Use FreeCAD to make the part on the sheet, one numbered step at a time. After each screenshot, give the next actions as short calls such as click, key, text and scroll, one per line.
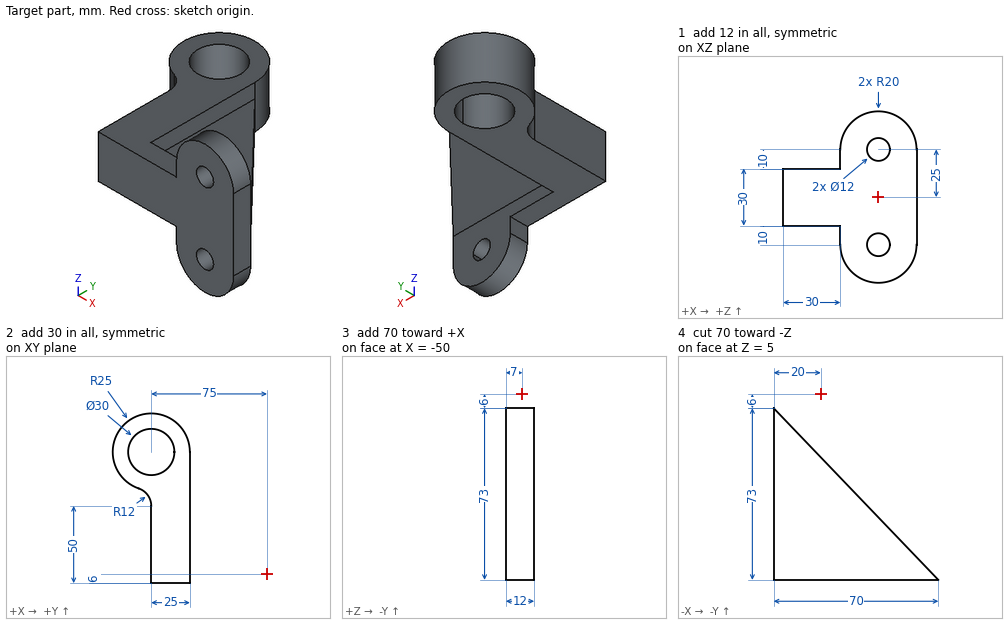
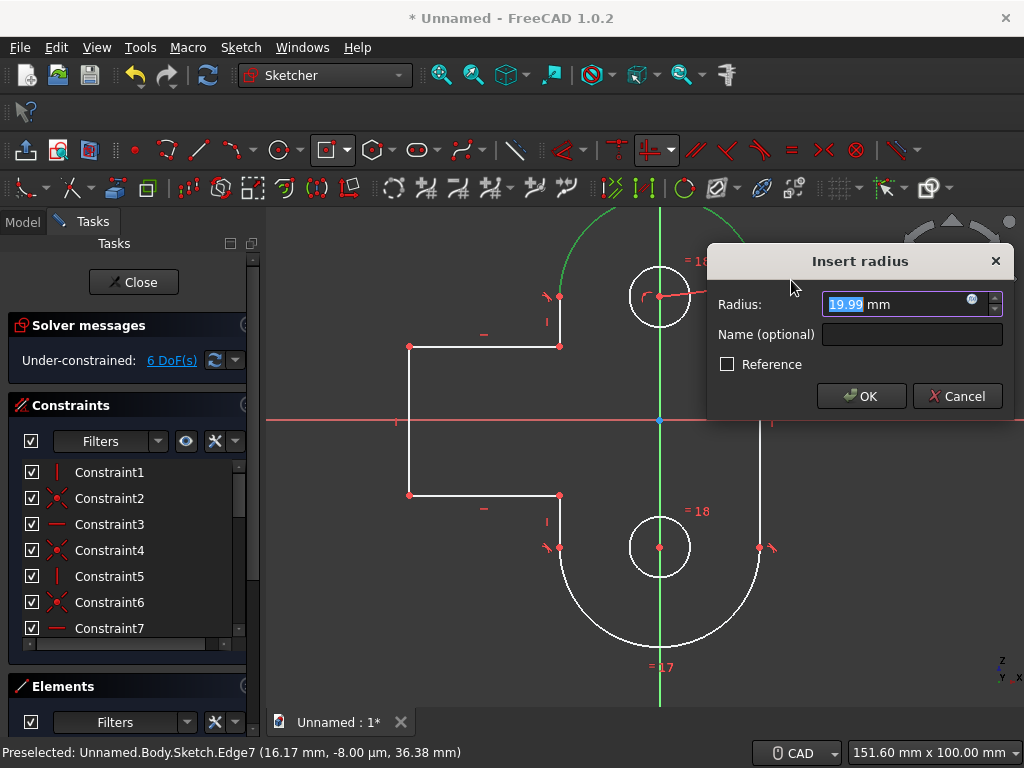
text(20)
key(Return)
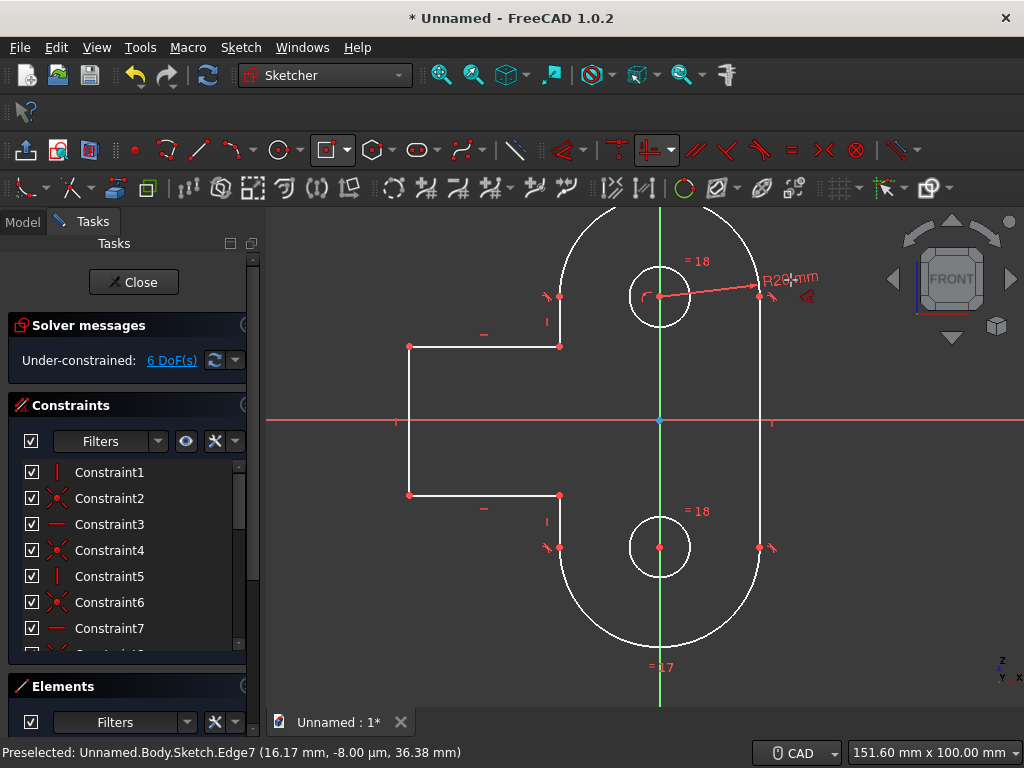
click(681, 275)
click(703, 252)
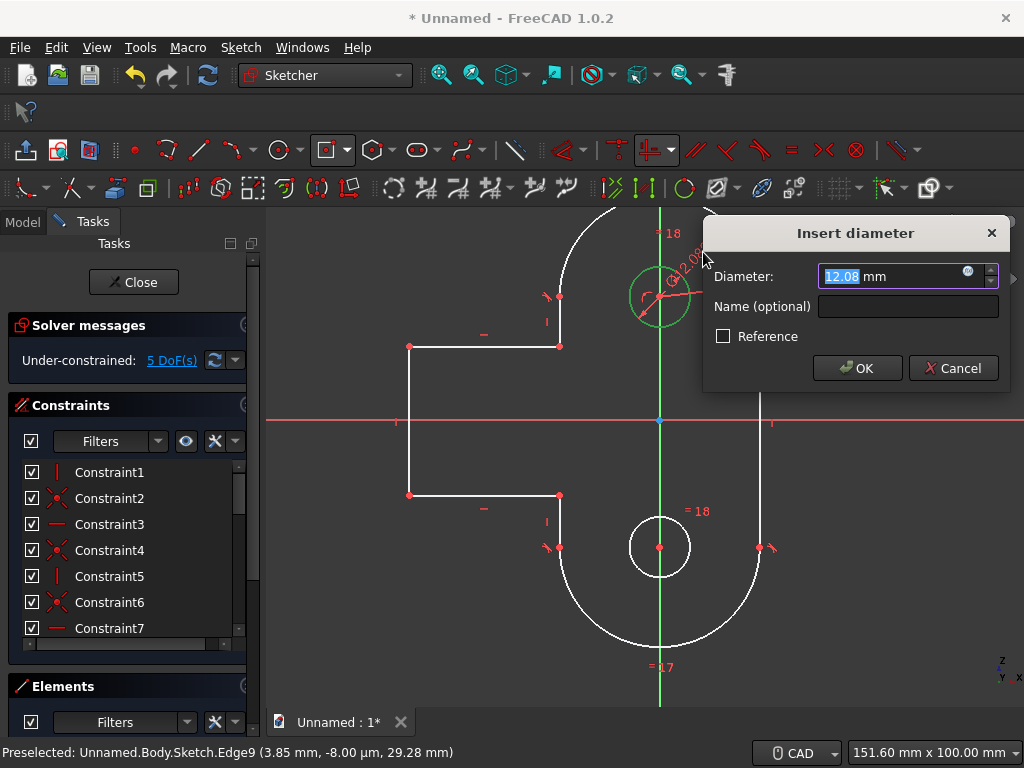
text(12)
key(Return)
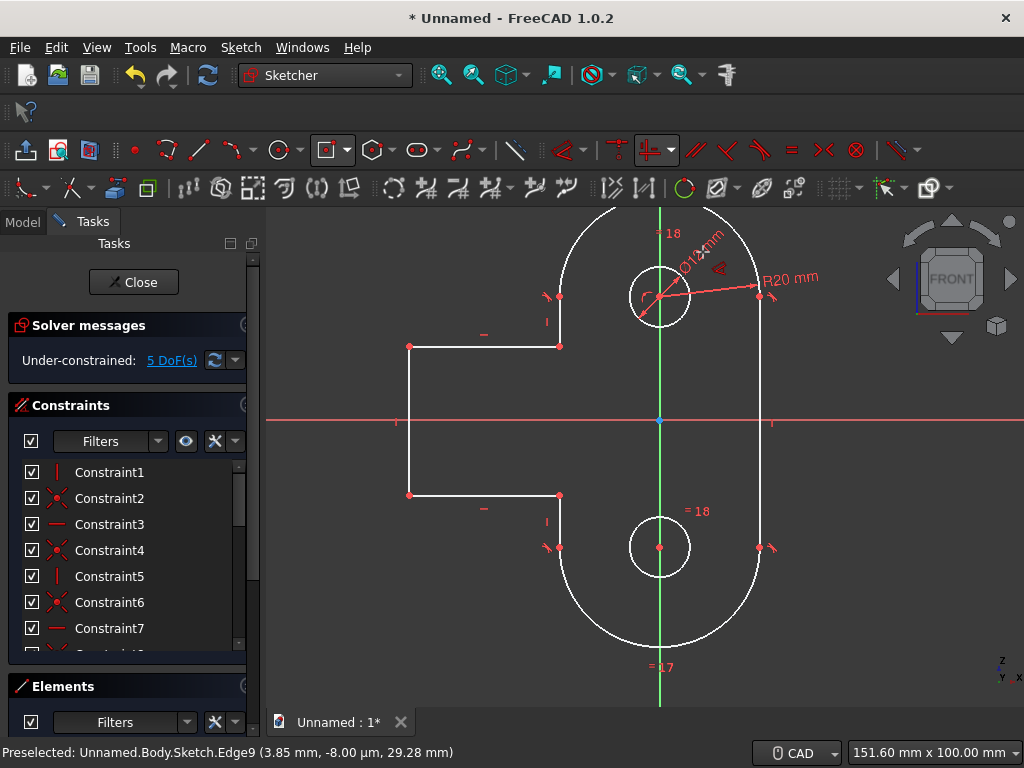
click(560, 532)
click(526, 522)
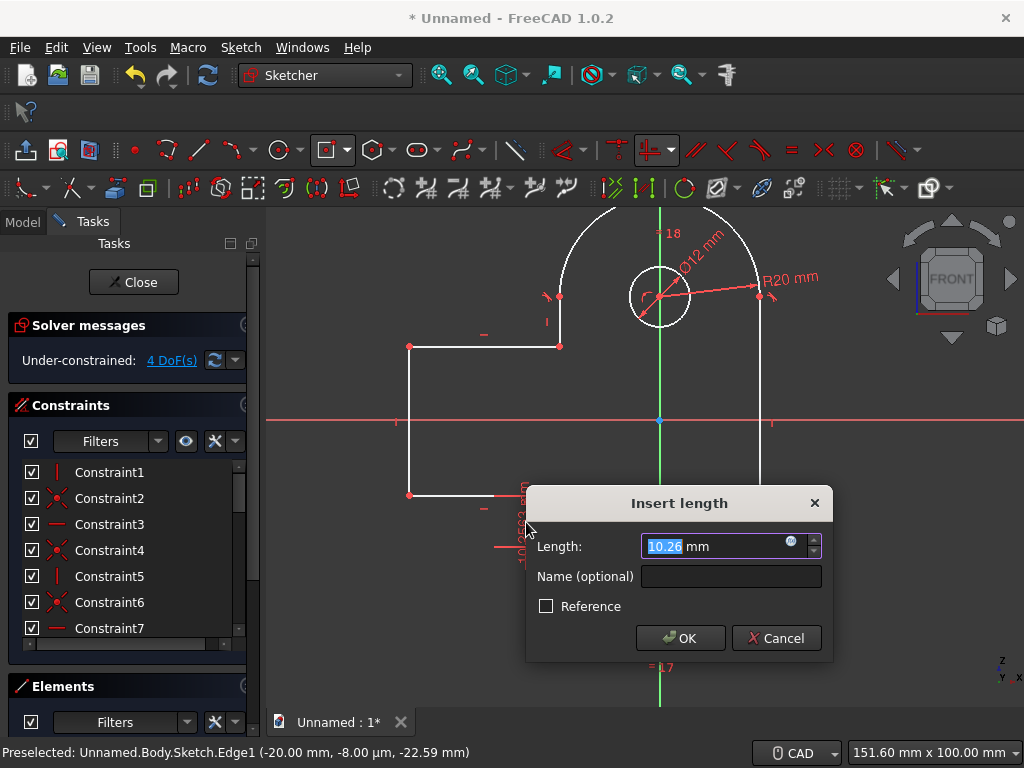
text(10)
key(Return)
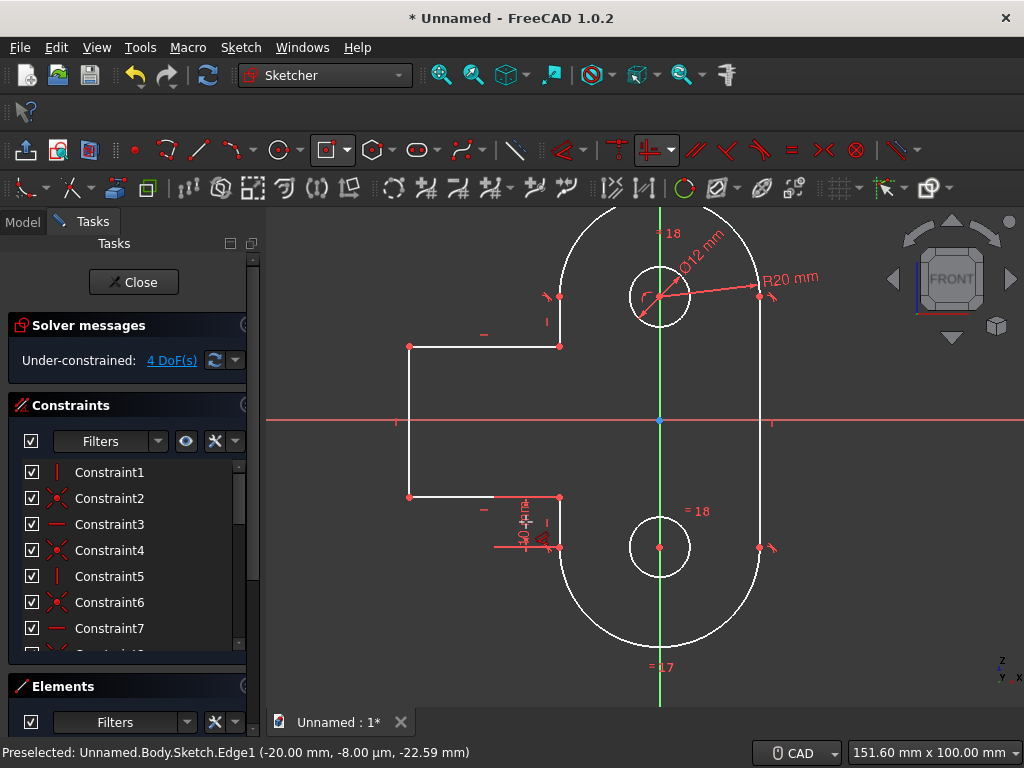
click(515, 497)
click(450, 531)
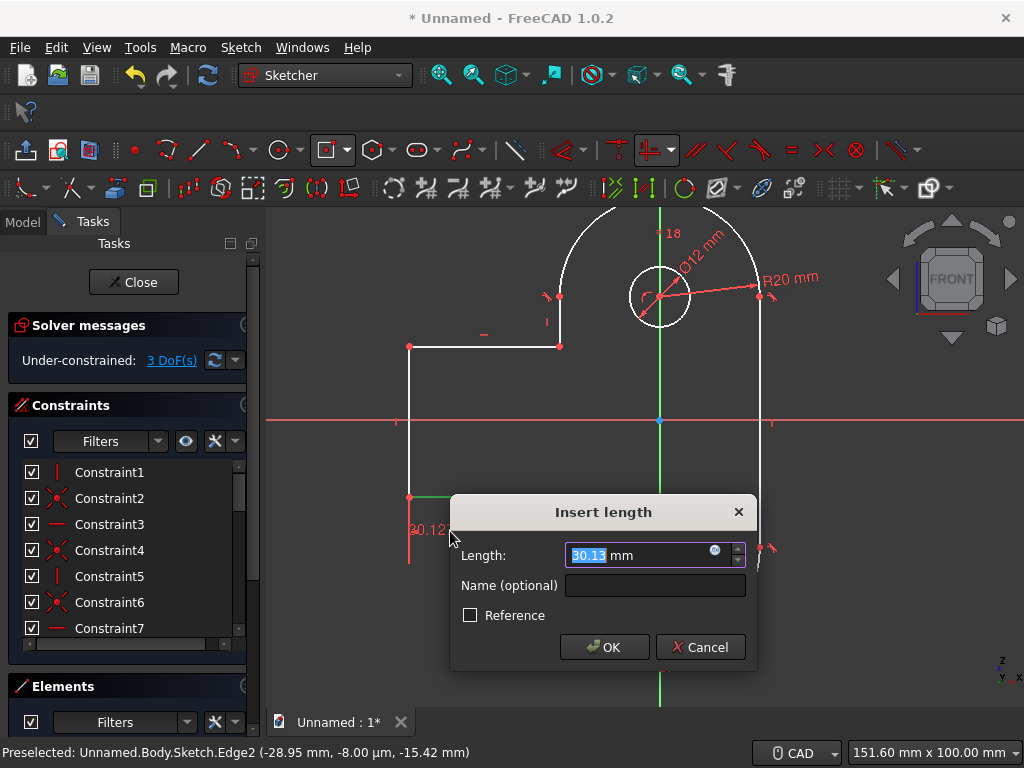
text(30)
key(Return)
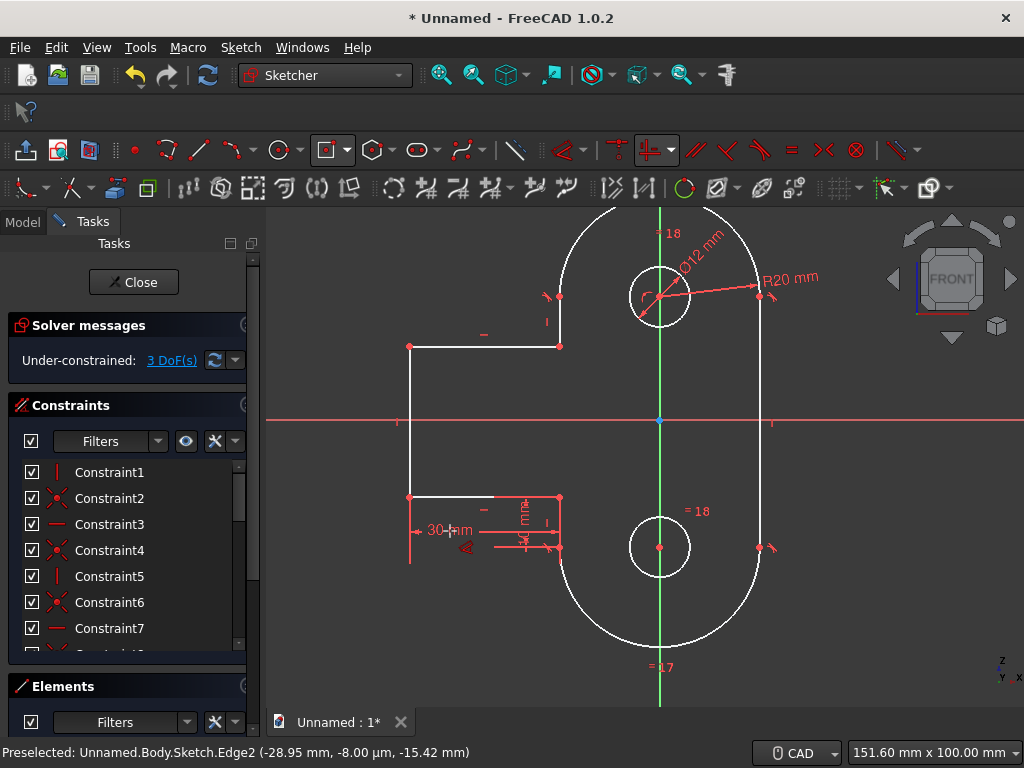
click(410, 452)
click(376, 387)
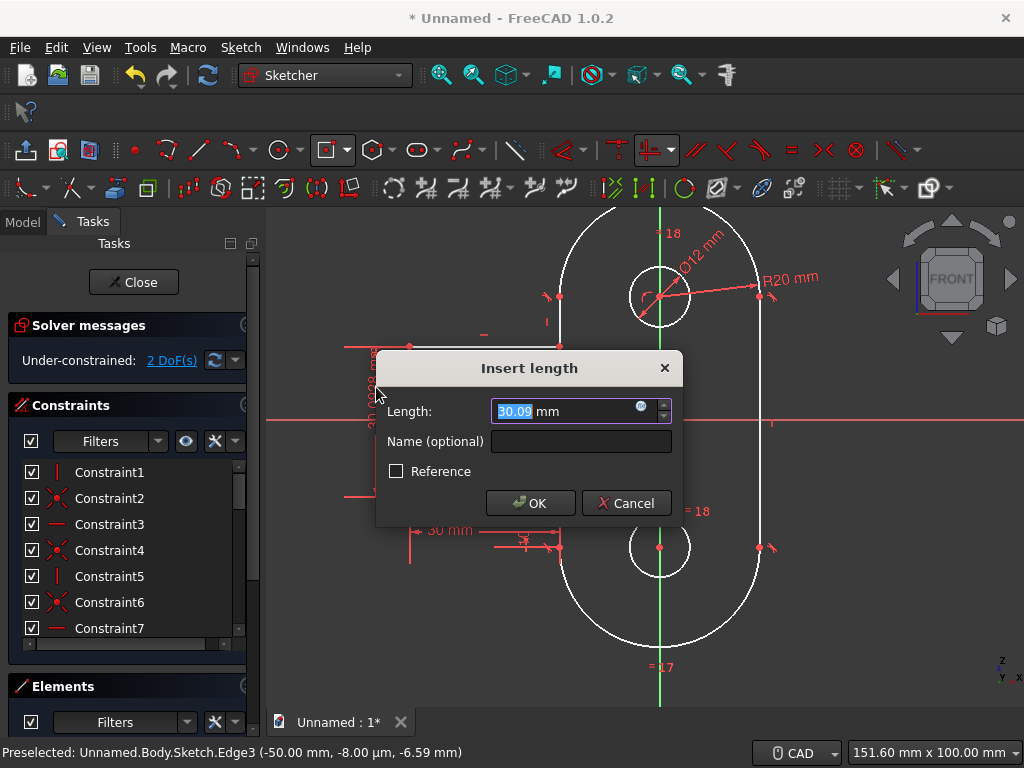
text(30)
key(Return)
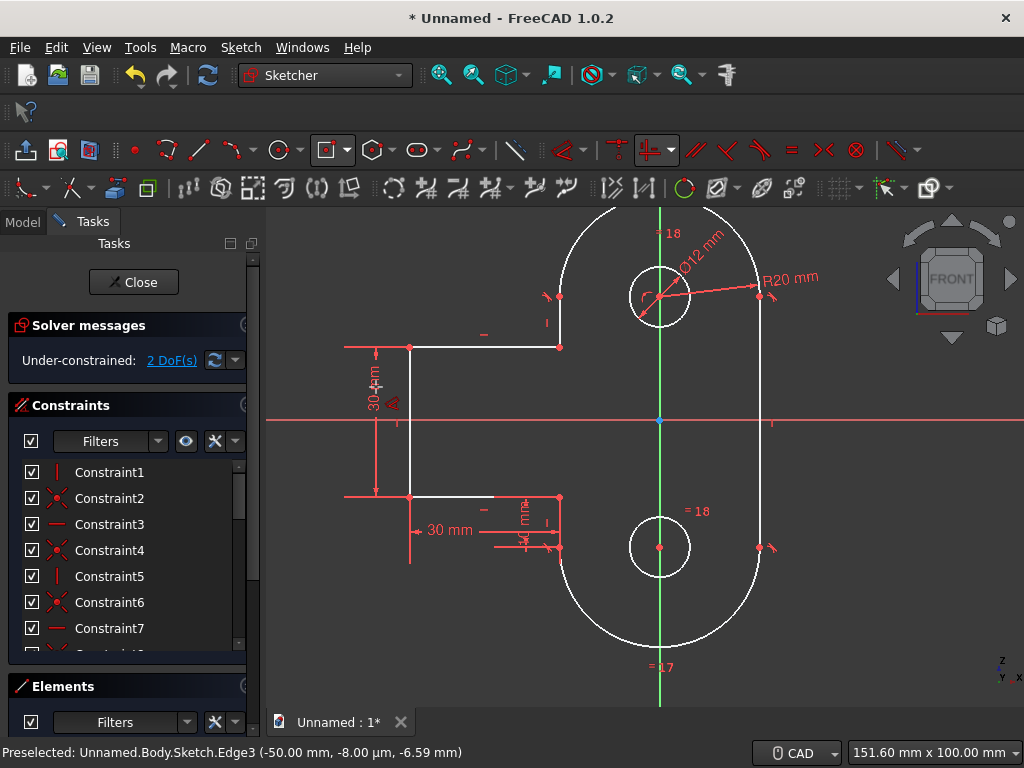
click(560, 332)
click(526, 322)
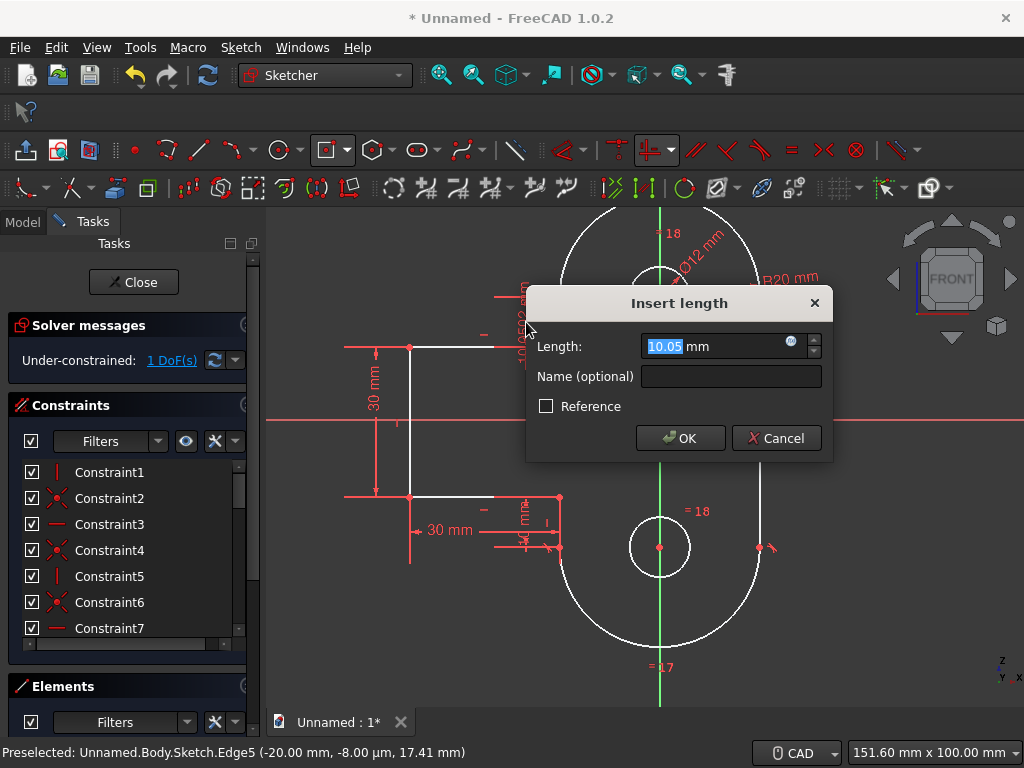
text(10)
key(Return)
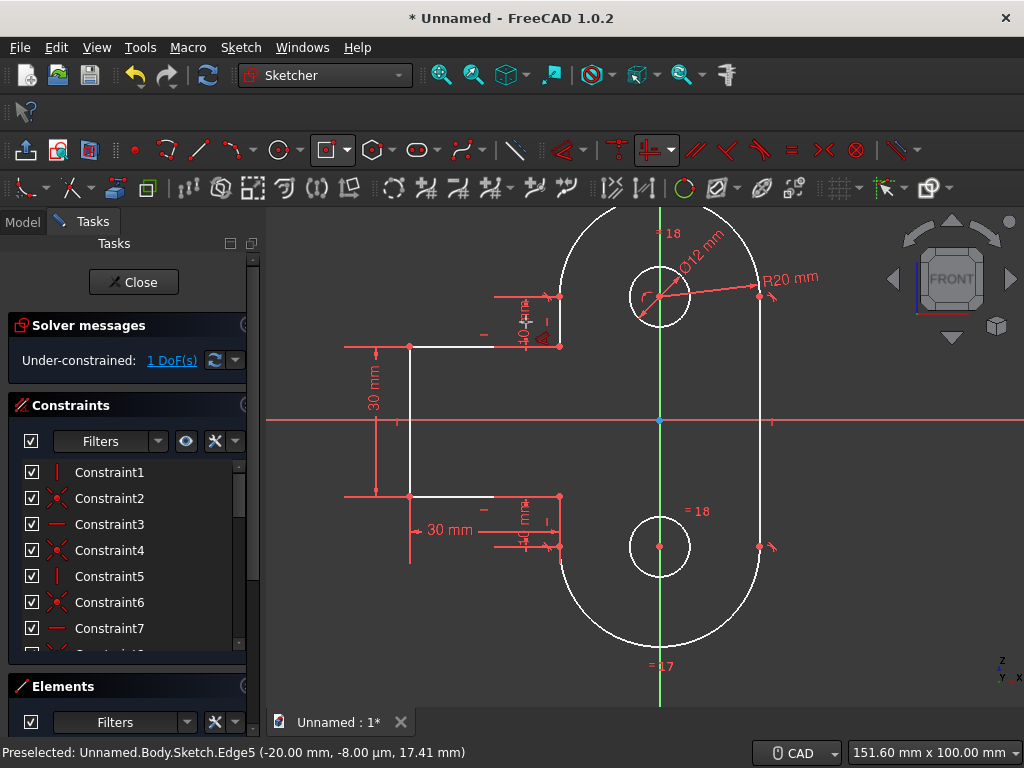
click(660, 297)
click(694, 358)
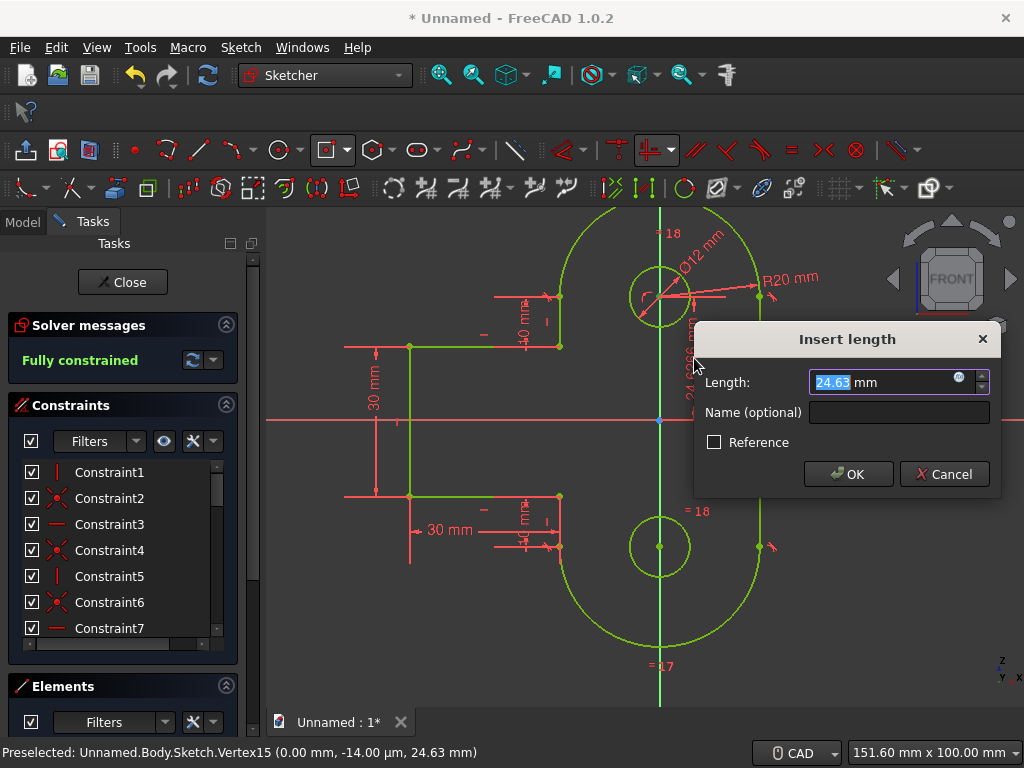
text(25)
key(Return)
key(Escape)